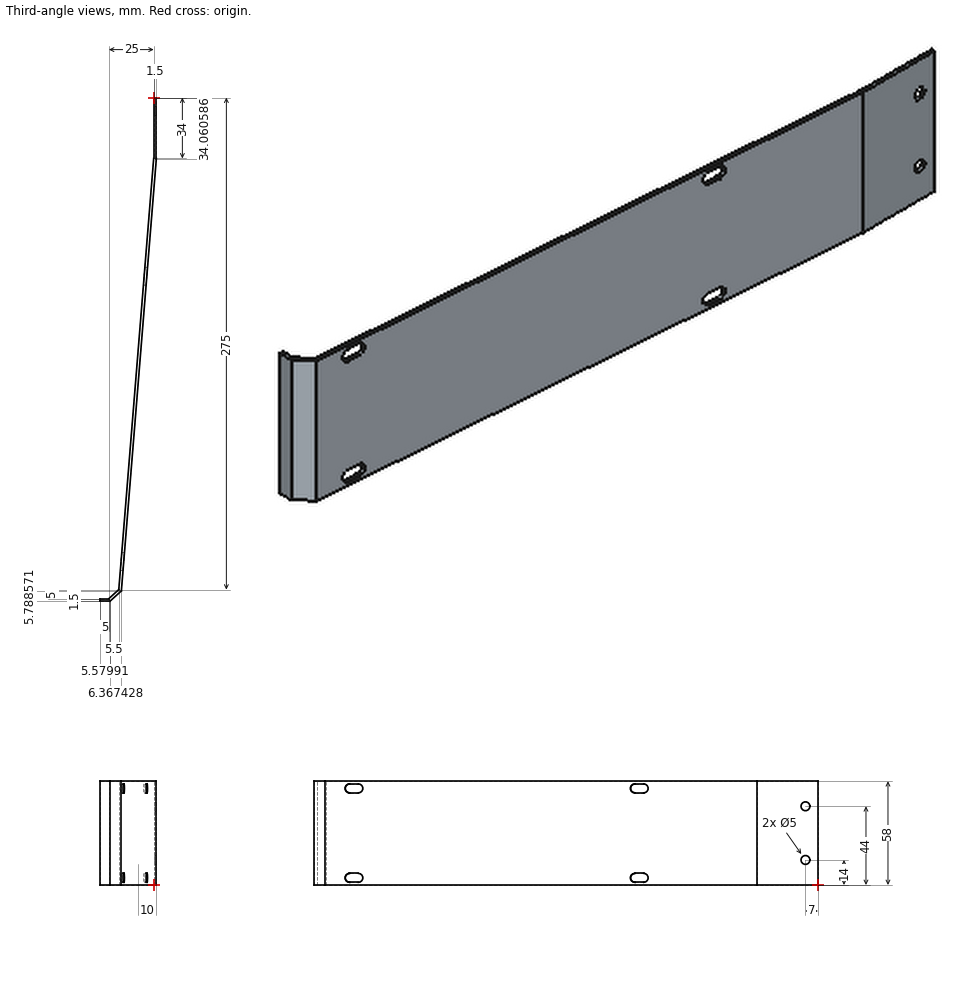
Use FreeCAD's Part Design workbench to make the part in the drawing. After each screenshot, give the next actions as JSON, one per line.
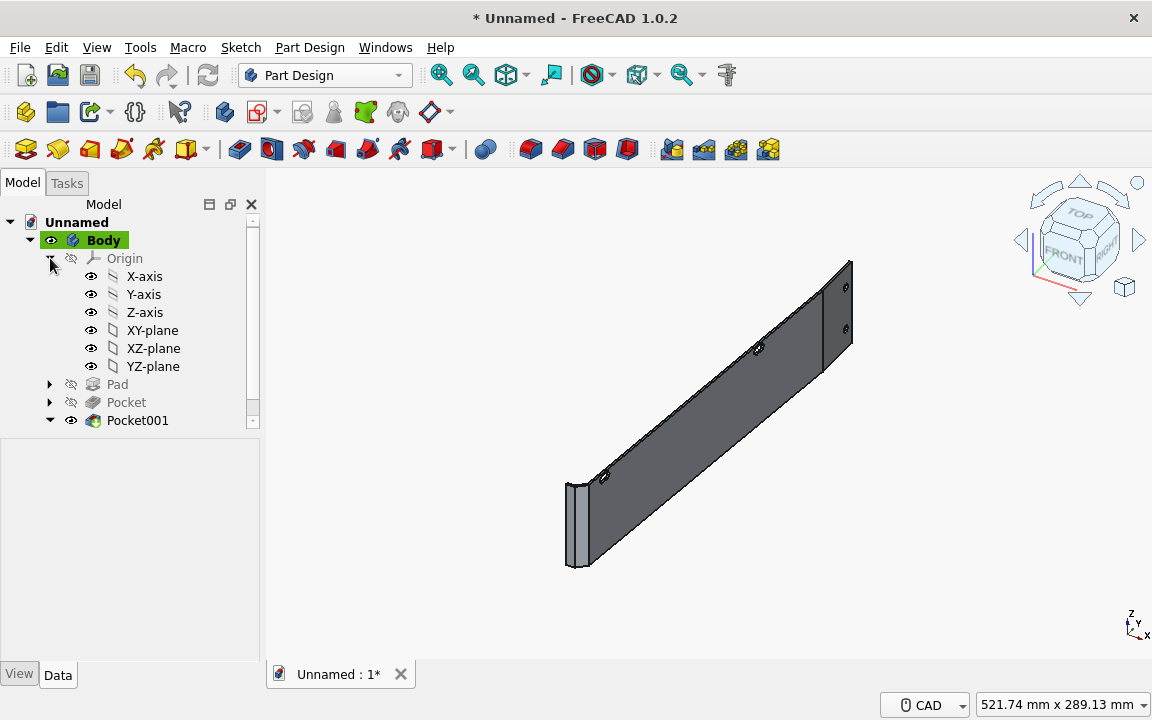
{"action": "left_click", "coordinate": [136, 330]}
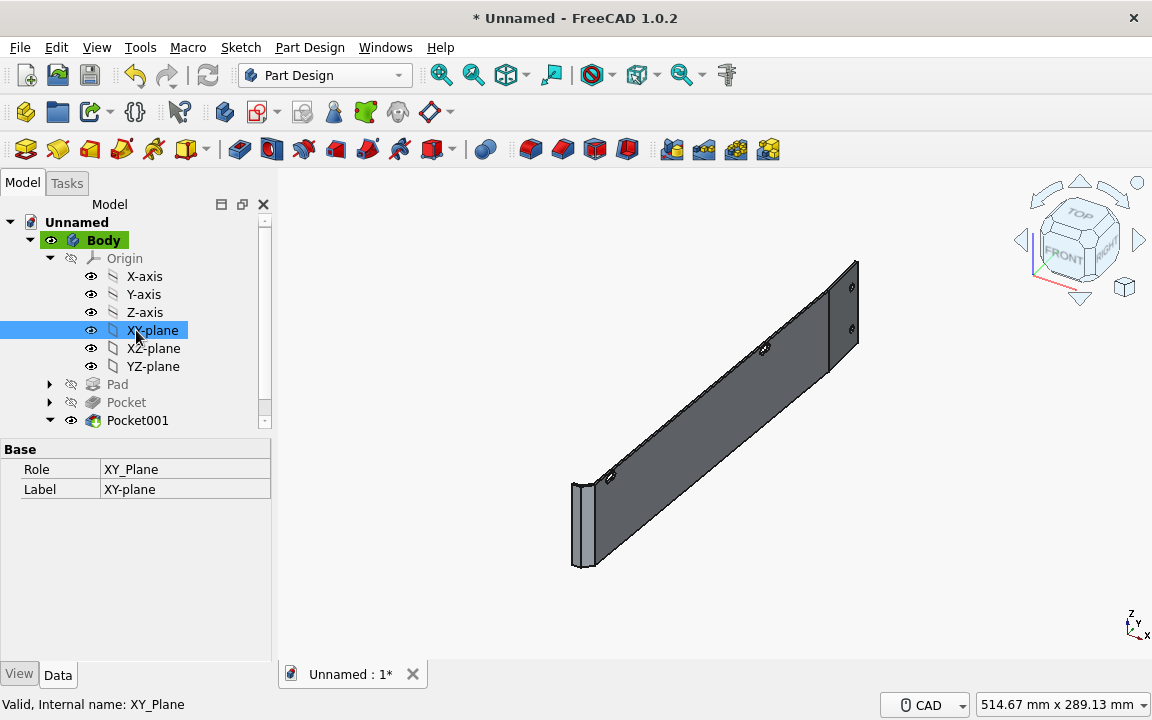
{"action": "left_click", "coordinate": [430, 112]}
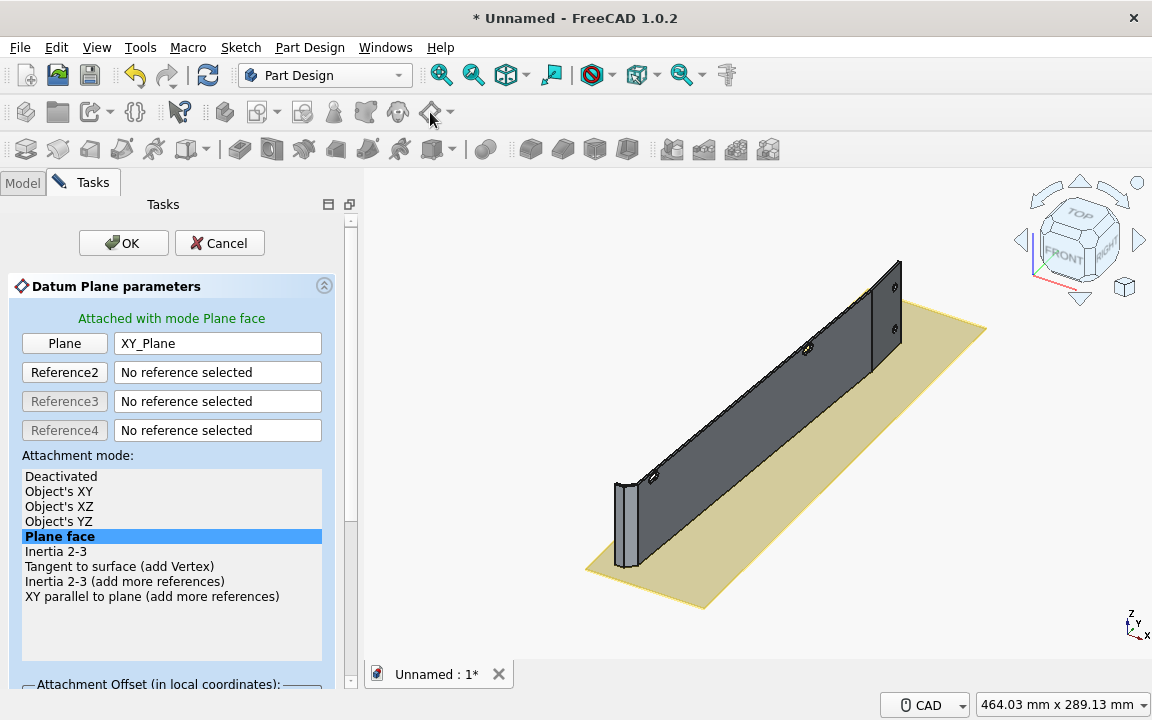
{"action": "scroll", "coordinate": [351, 451], "scroll_direction": "down", "scroll_amount": 3}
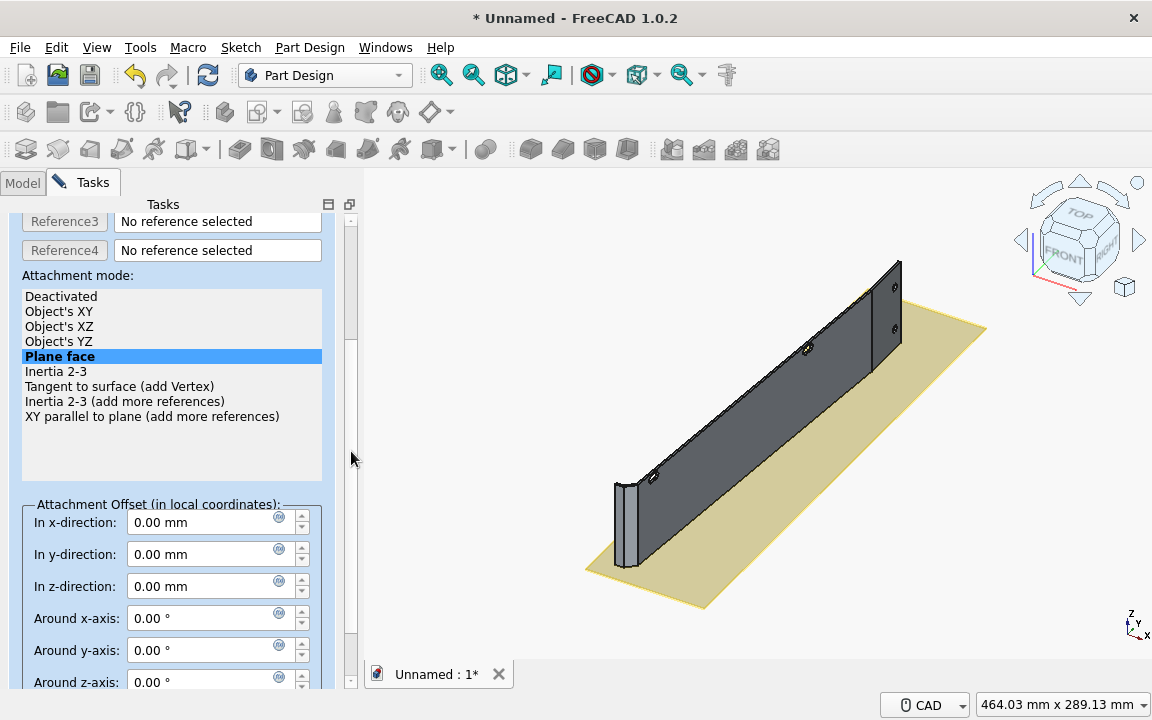
{"action": "triple_click", "coordinate": [210, 586]}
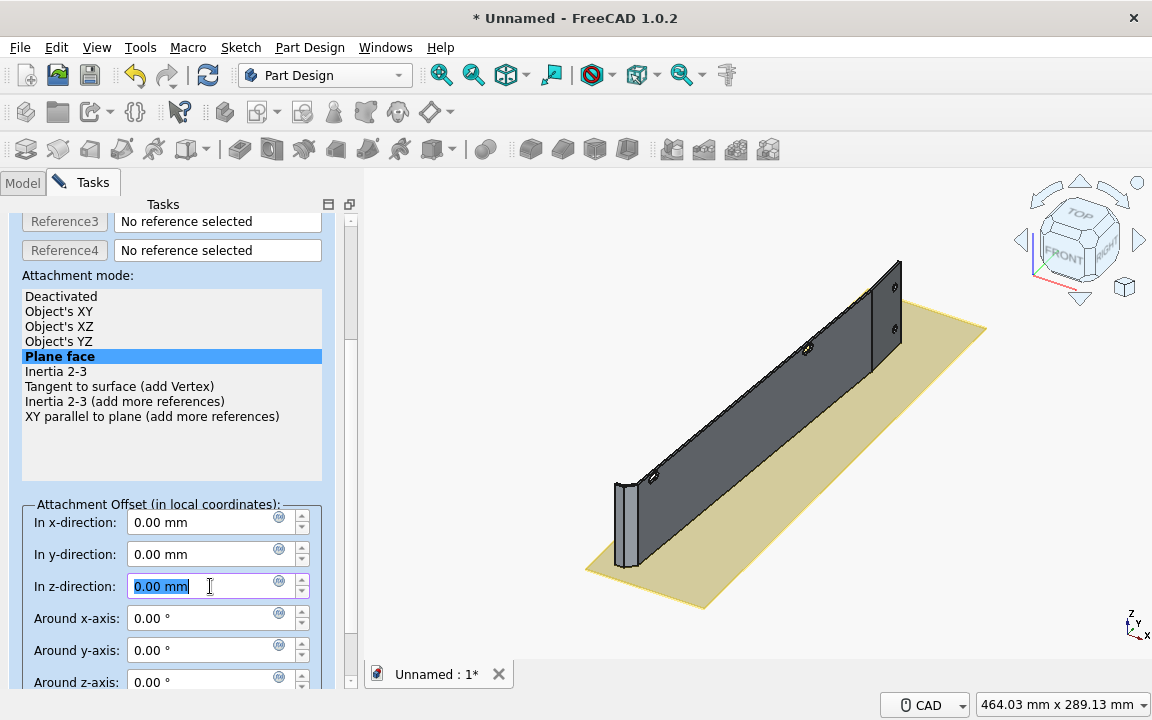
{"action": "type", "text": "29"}
{"action": "key", "text": "Tab"}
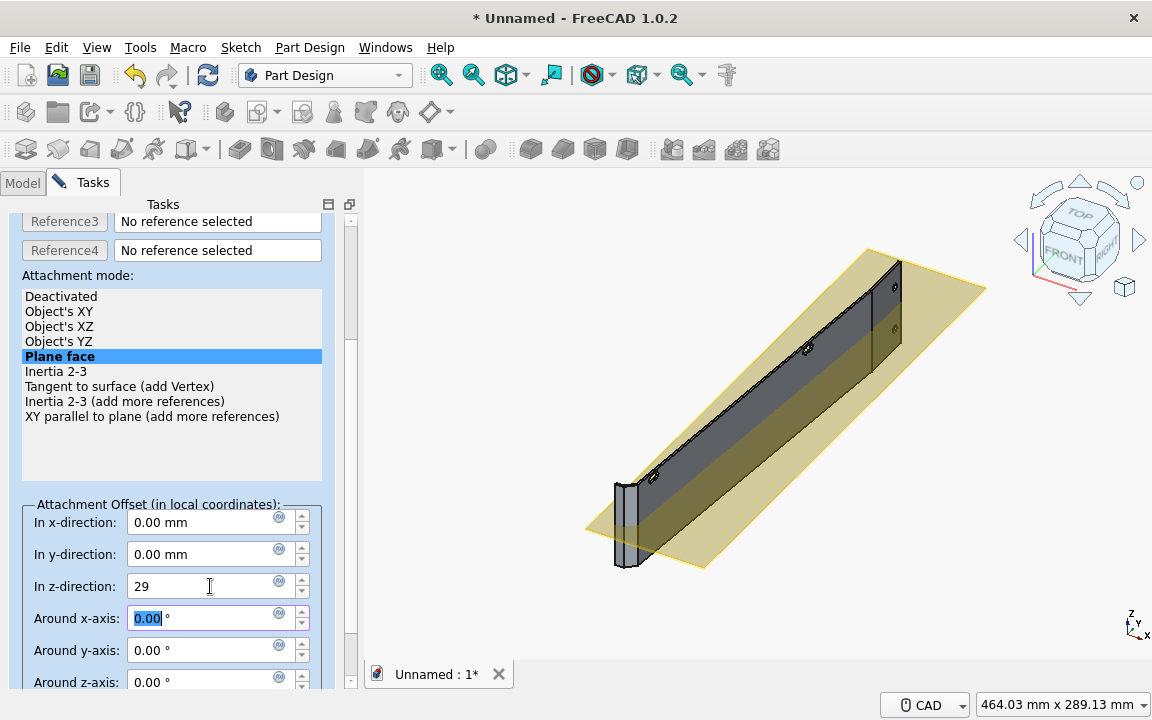
{"action": "scroll", "coordinate": [351, 451], "scroll_direction": "up", "scroll_amount": 4}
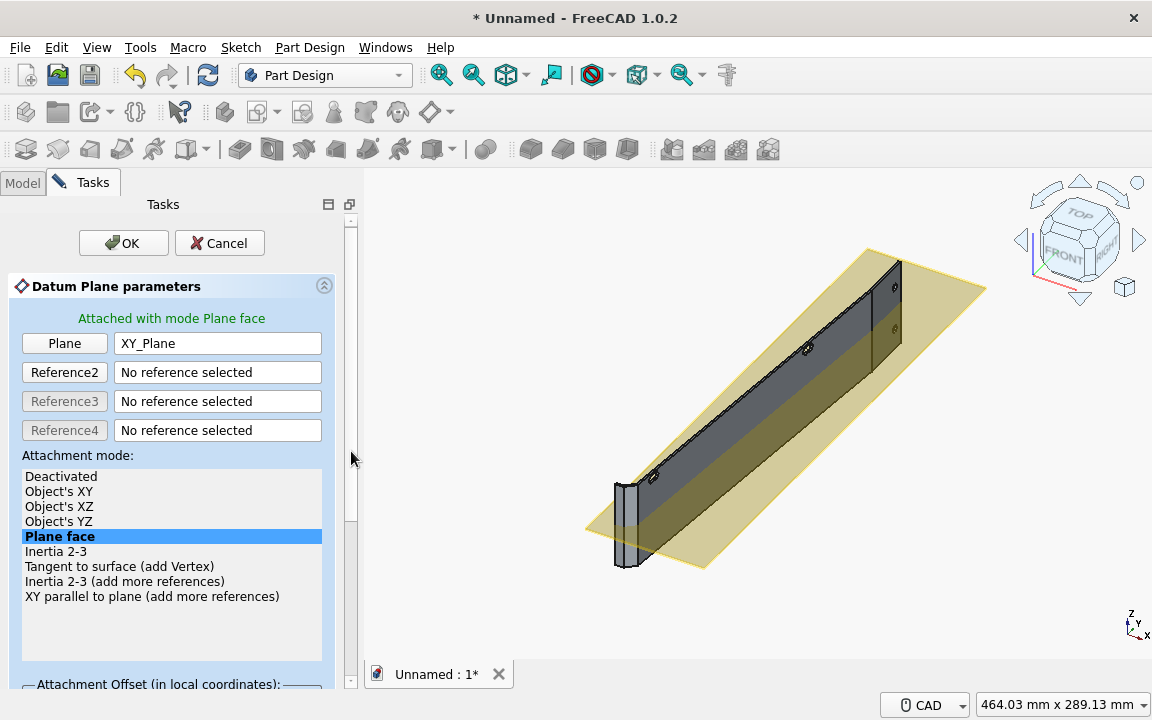
{"action": "left_click", "coordinate": [124, 243]}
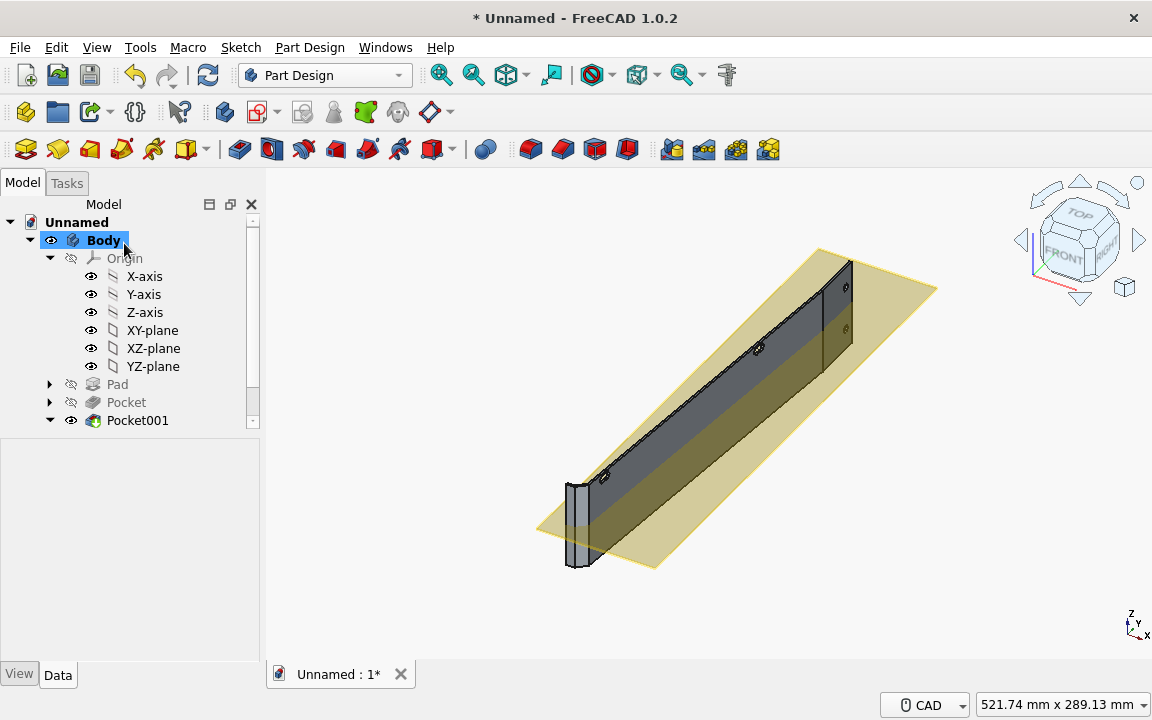
{"action": "left_click", "coordinate": [116, 420]}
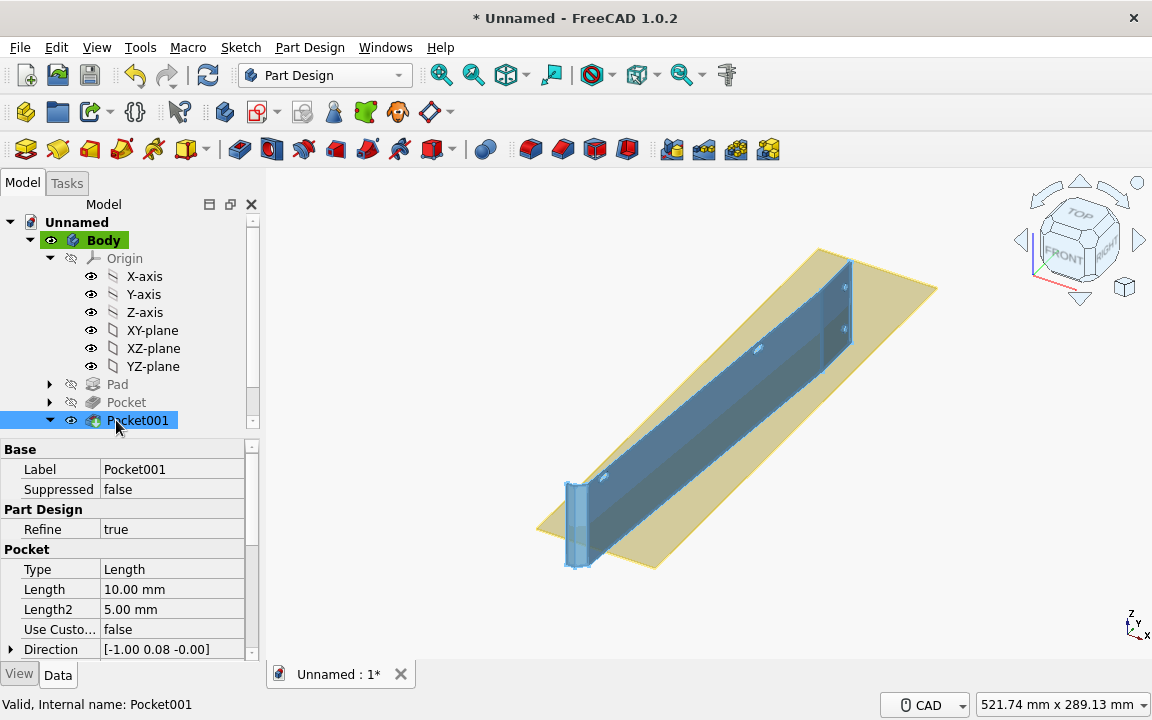
{"action": "left_click", "coordinate": [672, 150]}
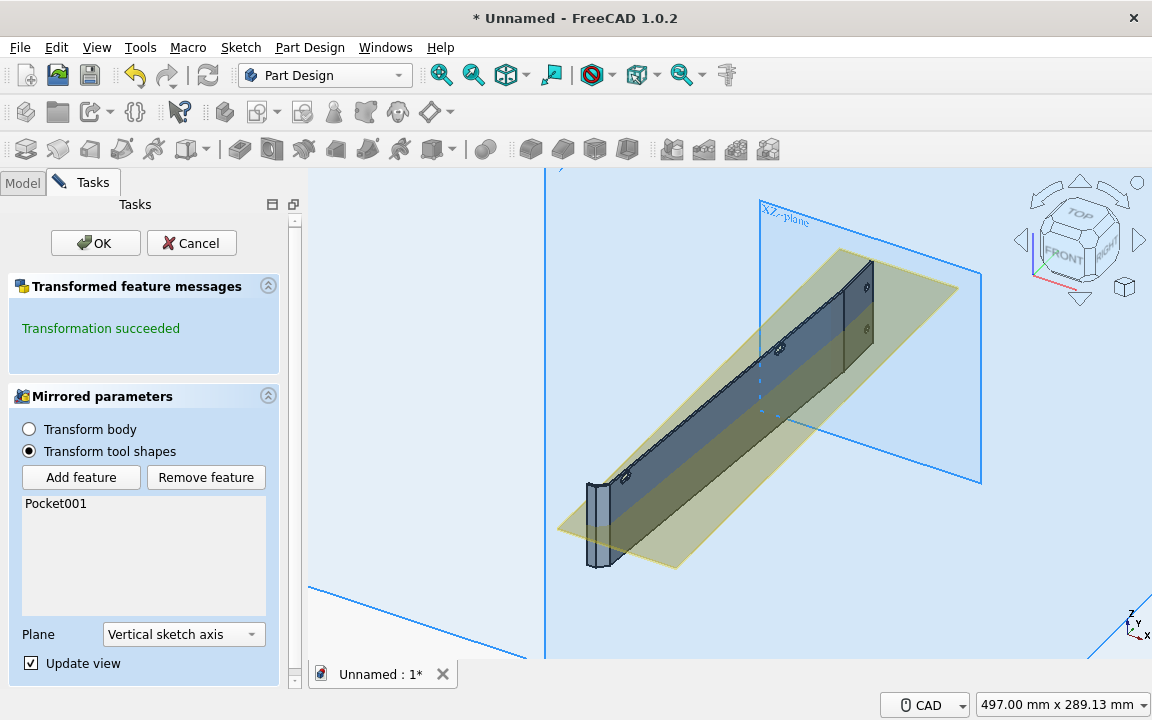
{"action": "left_click", "coordinate": [184, 634]}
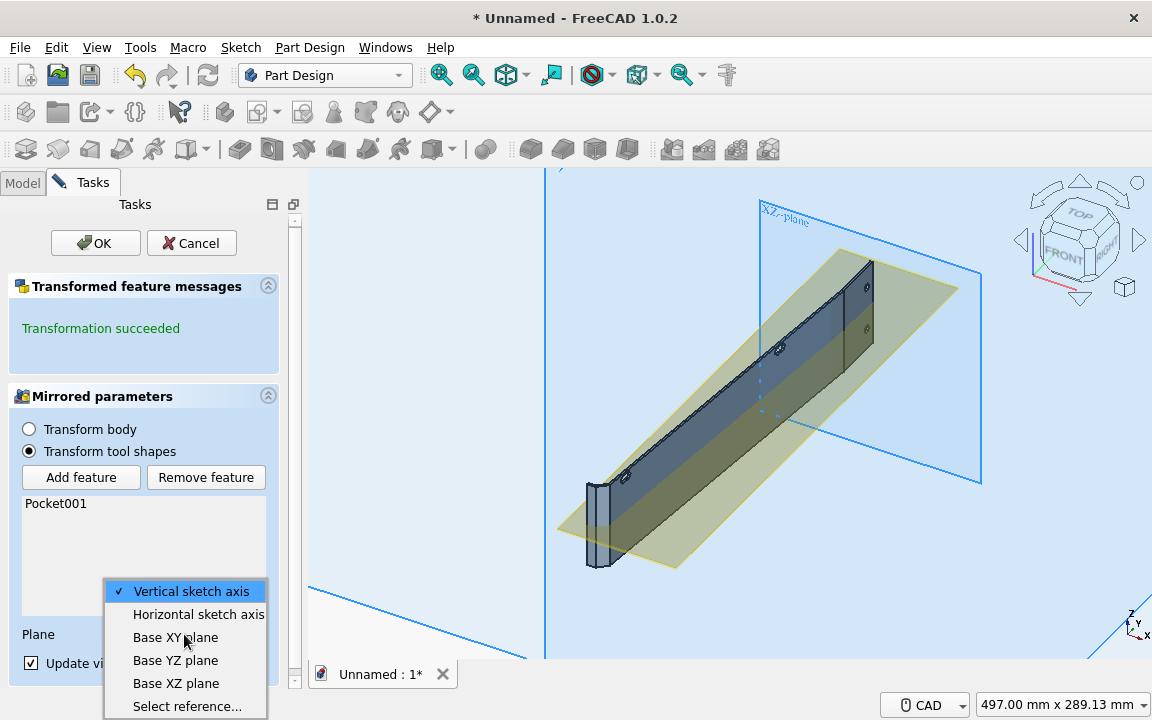
{"action": "left_click", "coordinate": [184, 706]}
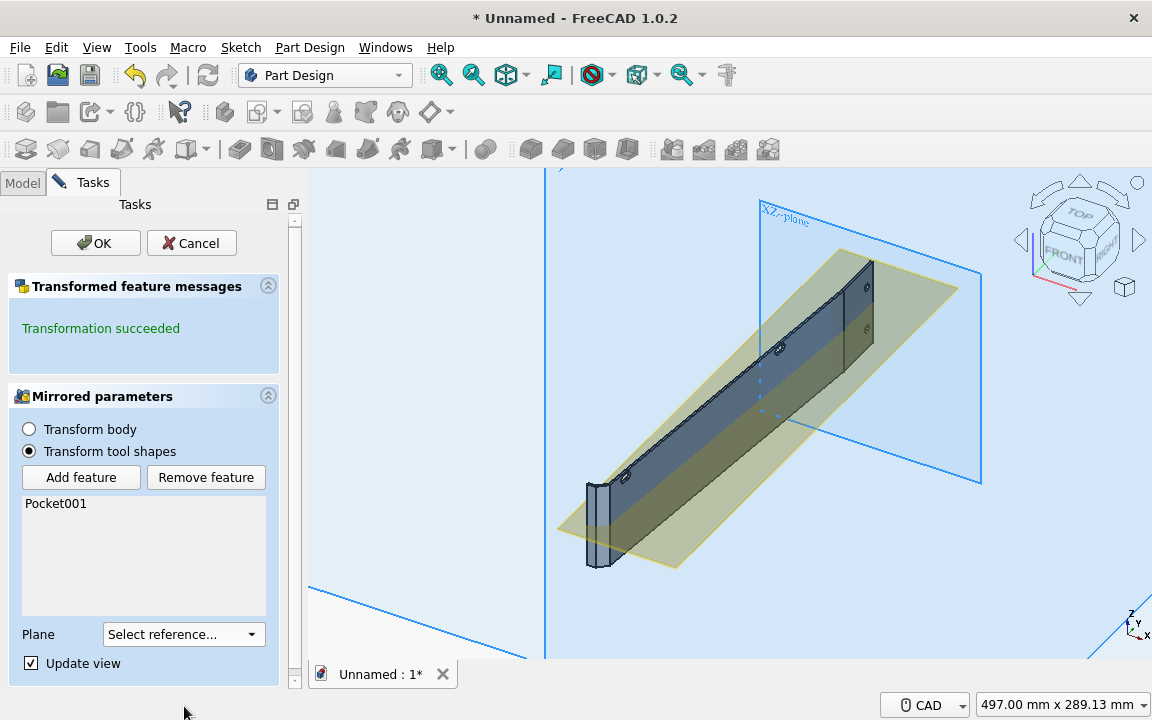
{"action": "left_click", "coordinate": [23, 182]}